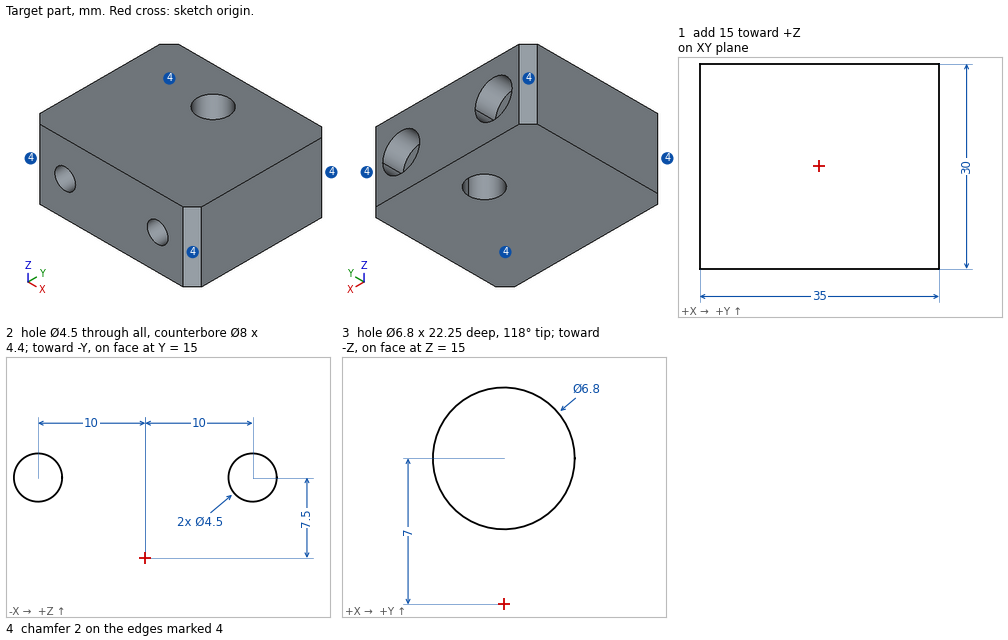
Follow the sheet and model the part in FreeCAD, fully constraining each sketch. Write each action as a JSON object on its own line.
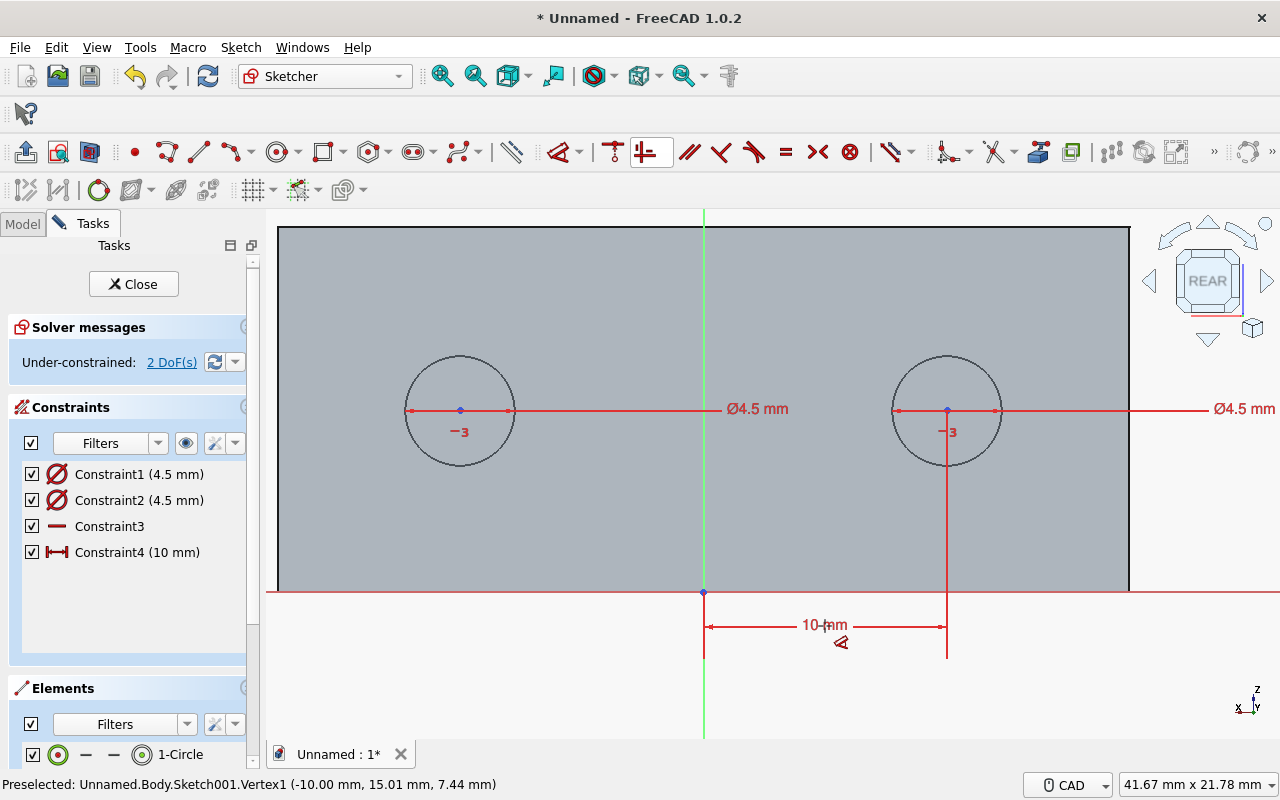
{"action": "left_click", "coordinate": [460, 411]}
{"action": "left_click", "coordinate": [582, 626]}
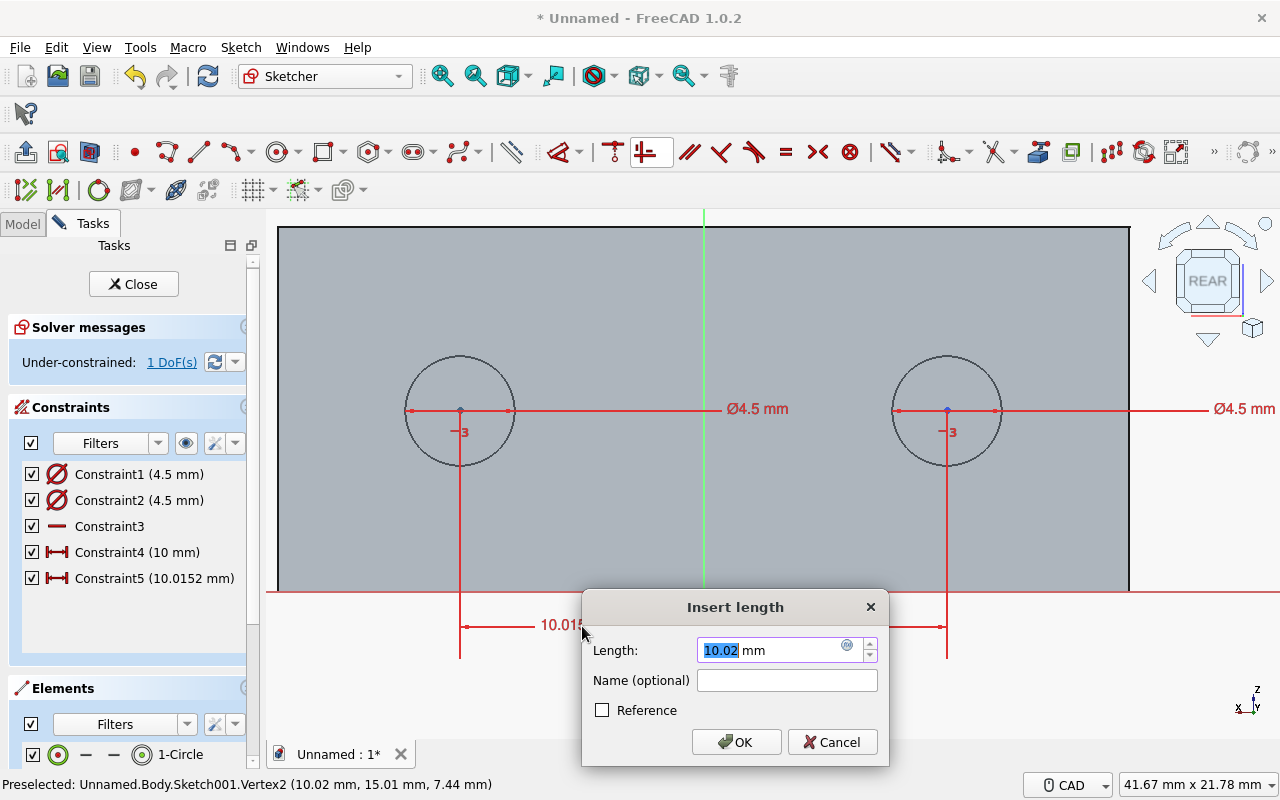
{"action": "type", "text": "10"}
{"action": "key", "text": "Return"}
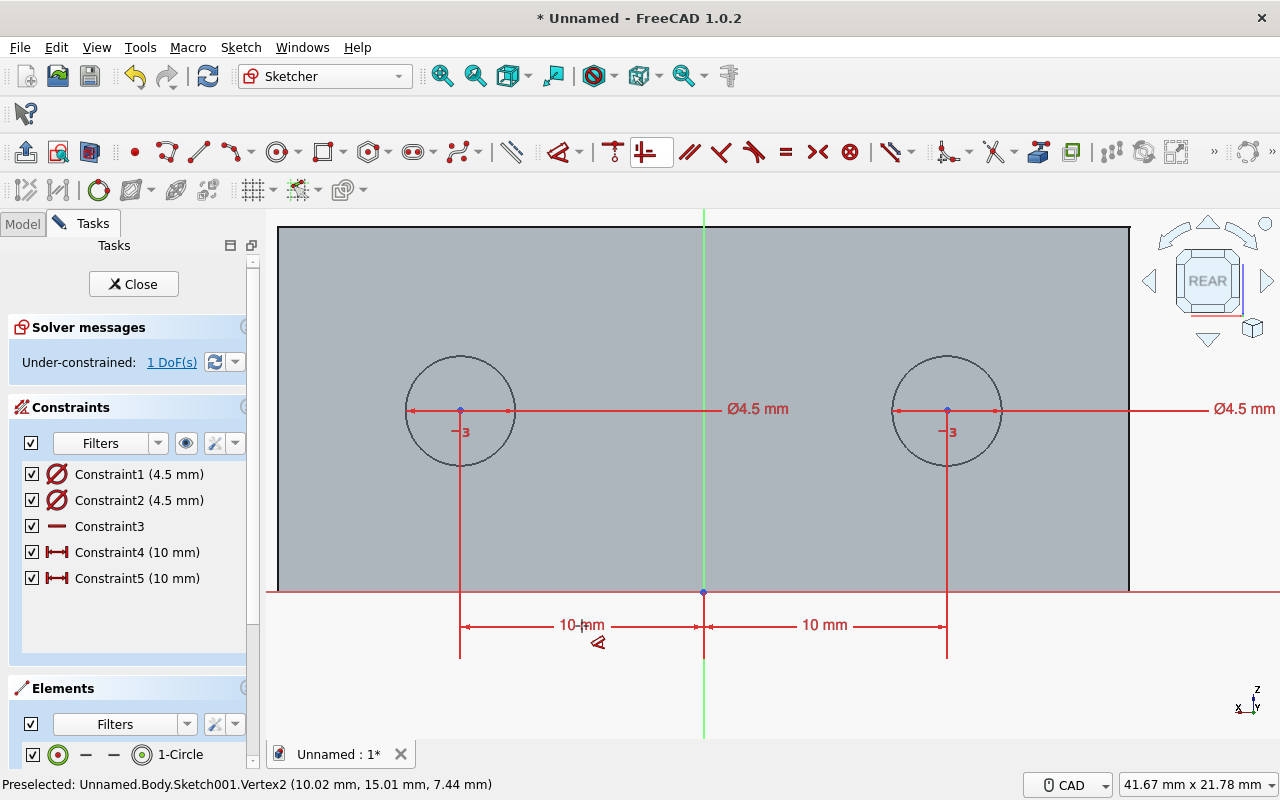
{"action": "left_click", "coordinate": [947, 411]}
{"action": "left_click", "coordinate": [981, 502]}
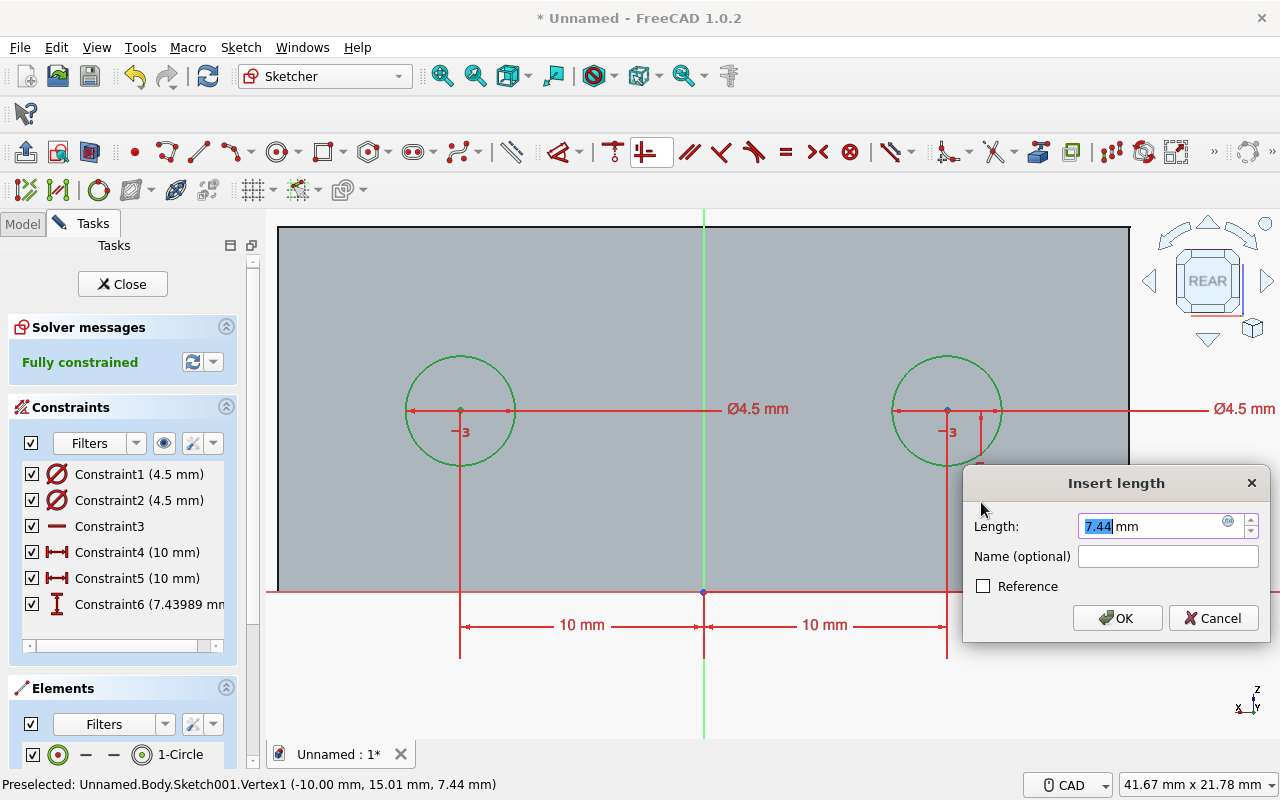
{"action": "type", "text": "7.5"}
{"action": "key", "text": "Return"}
{"action": "key", "text": "Escape"}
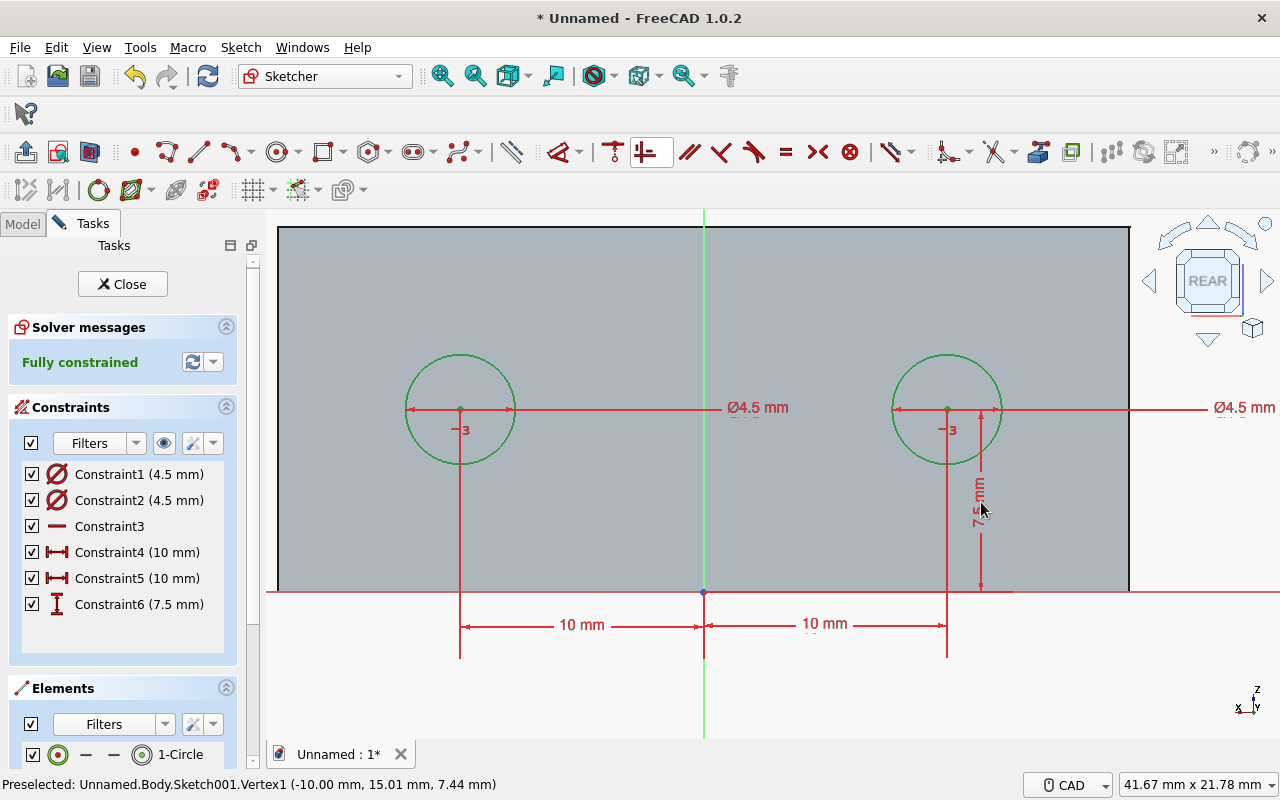
{"action": "left_click", "coordinate": [123, 284]}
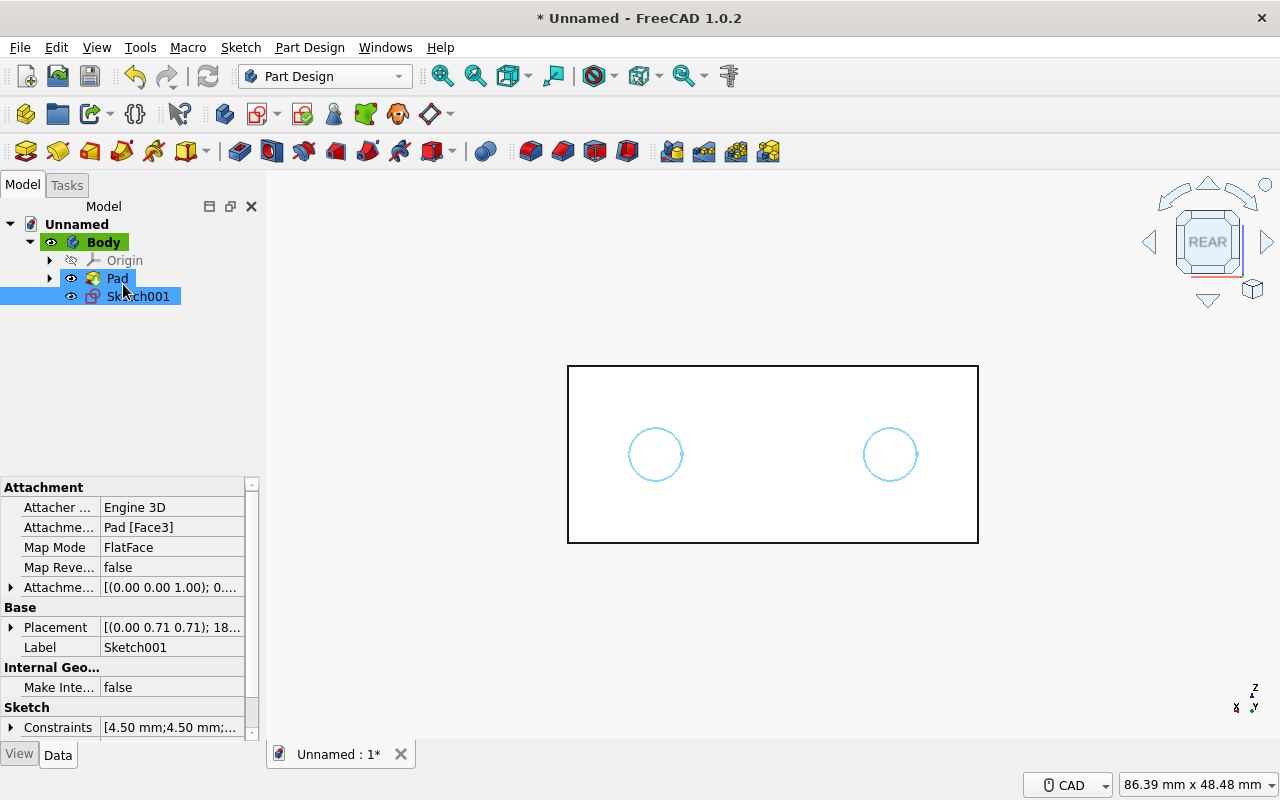
{"action": "left_click", "coordinate": [272, 152]}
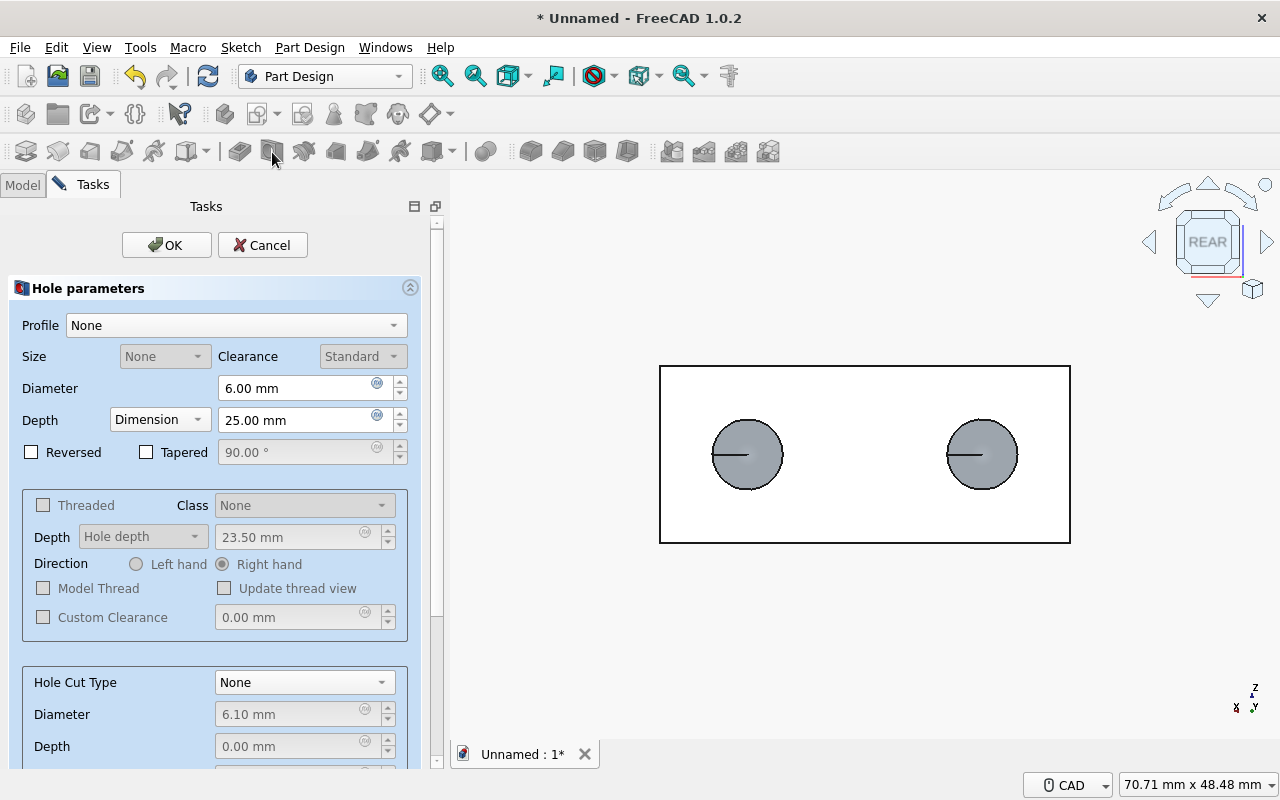
{"action": "triple_click", "coordinate": [305, 388]}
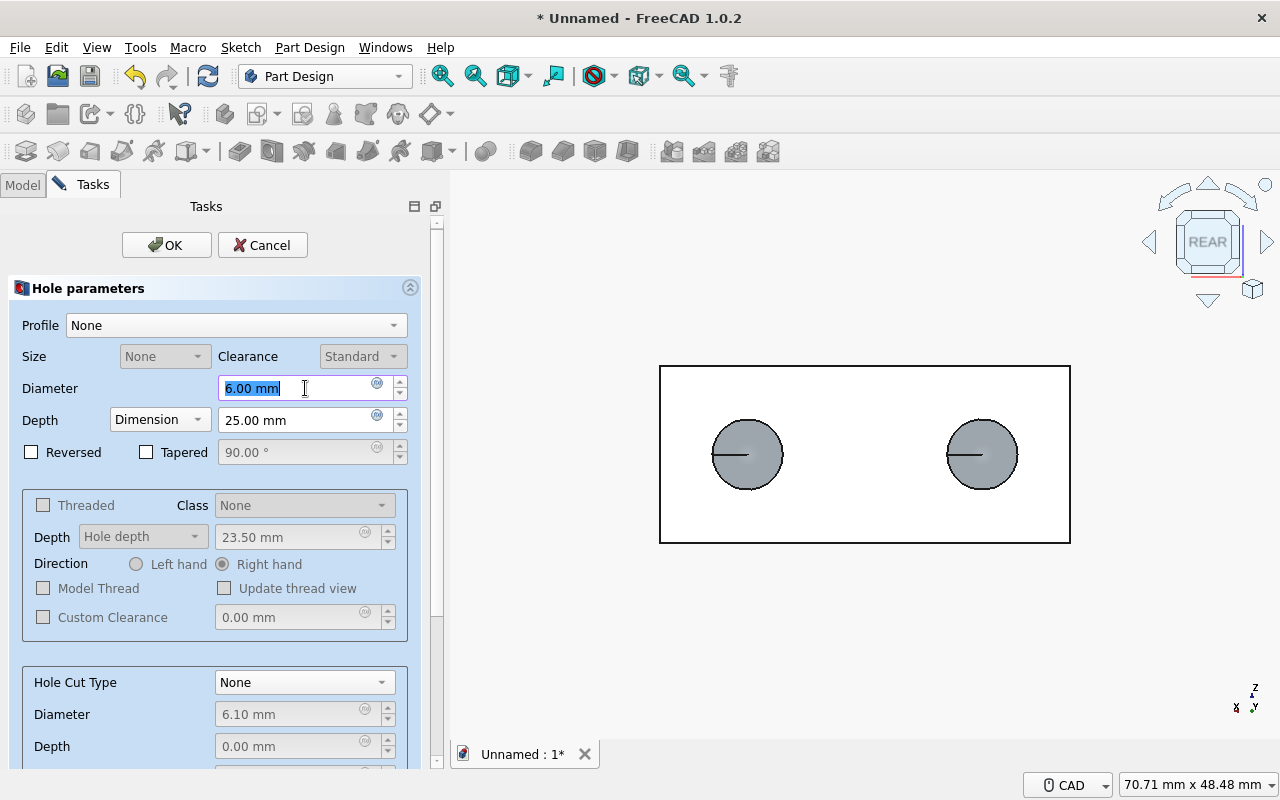
{"action": "type", "text": "4.5"}
{"action": "key", "text": "Tab"}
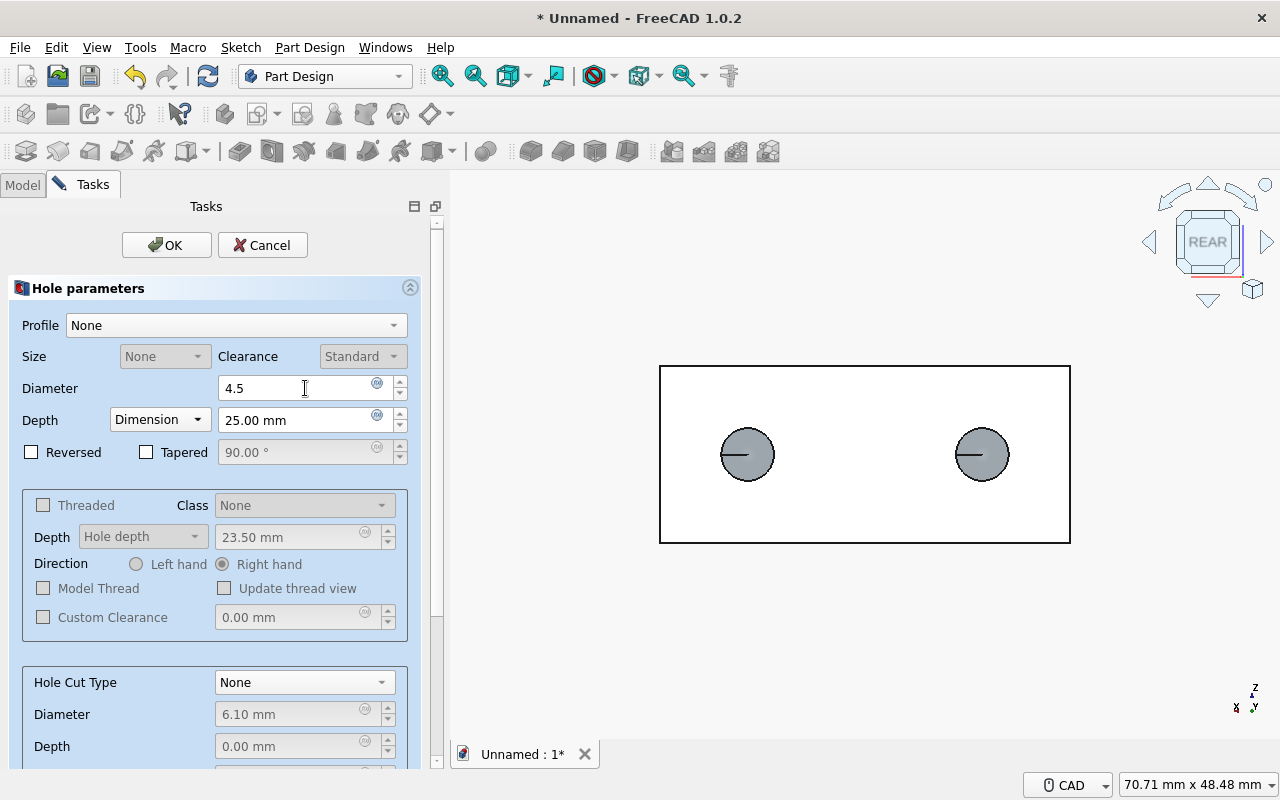
{"action": "left_click", "coordinate": [161, 420]}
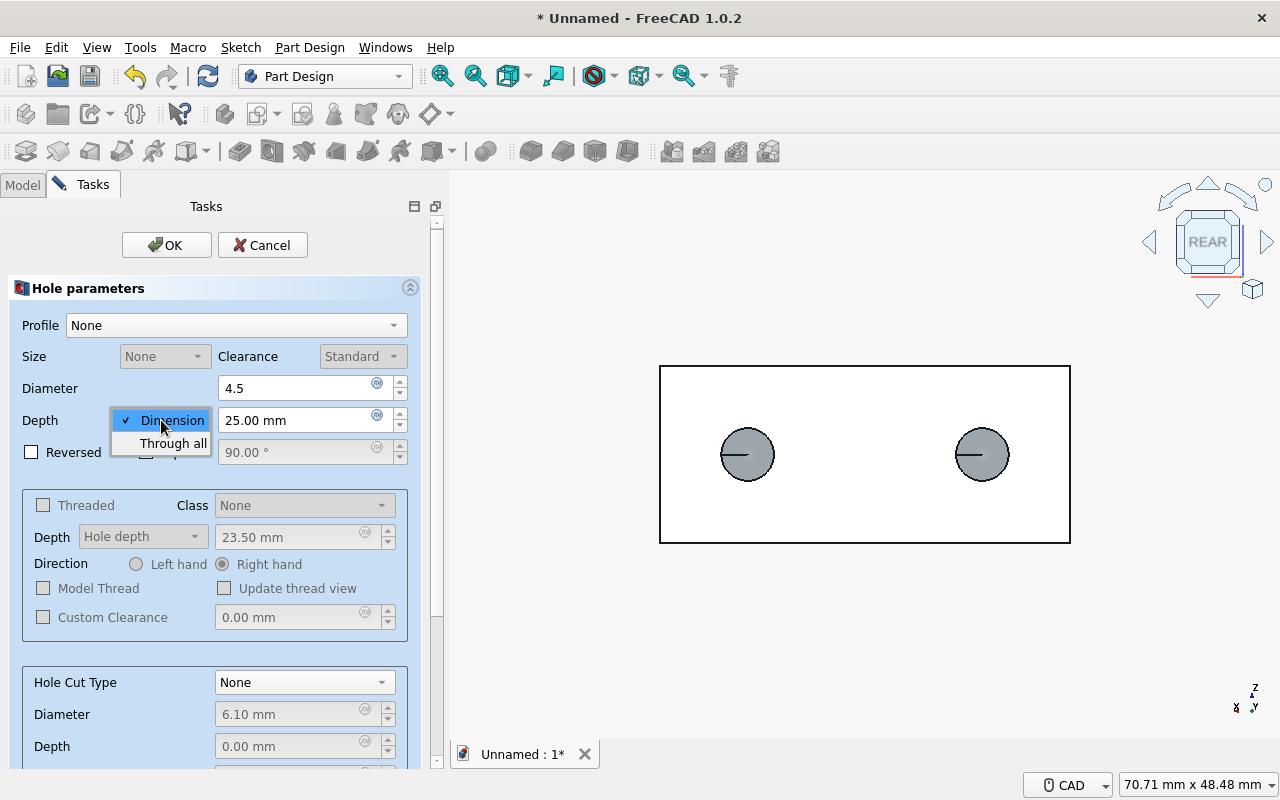
{"action": "left_click", "coordinate": [160, 444]}